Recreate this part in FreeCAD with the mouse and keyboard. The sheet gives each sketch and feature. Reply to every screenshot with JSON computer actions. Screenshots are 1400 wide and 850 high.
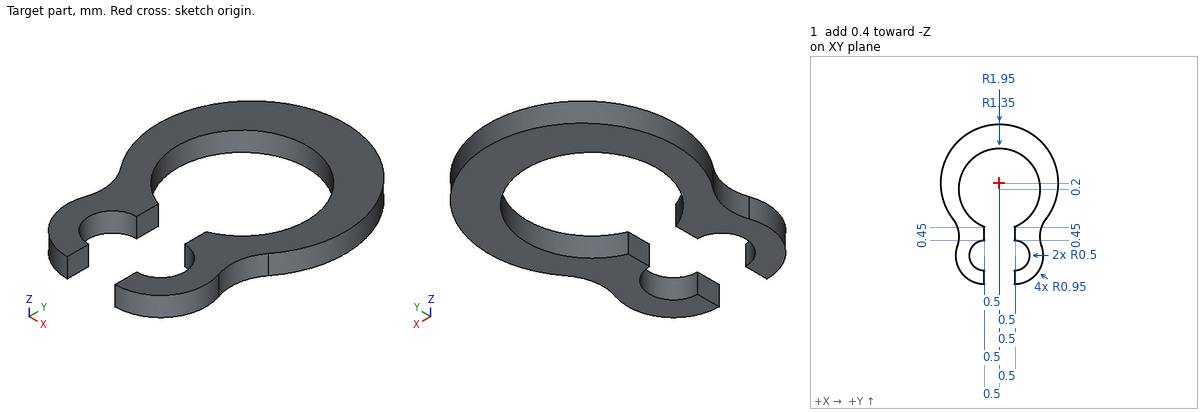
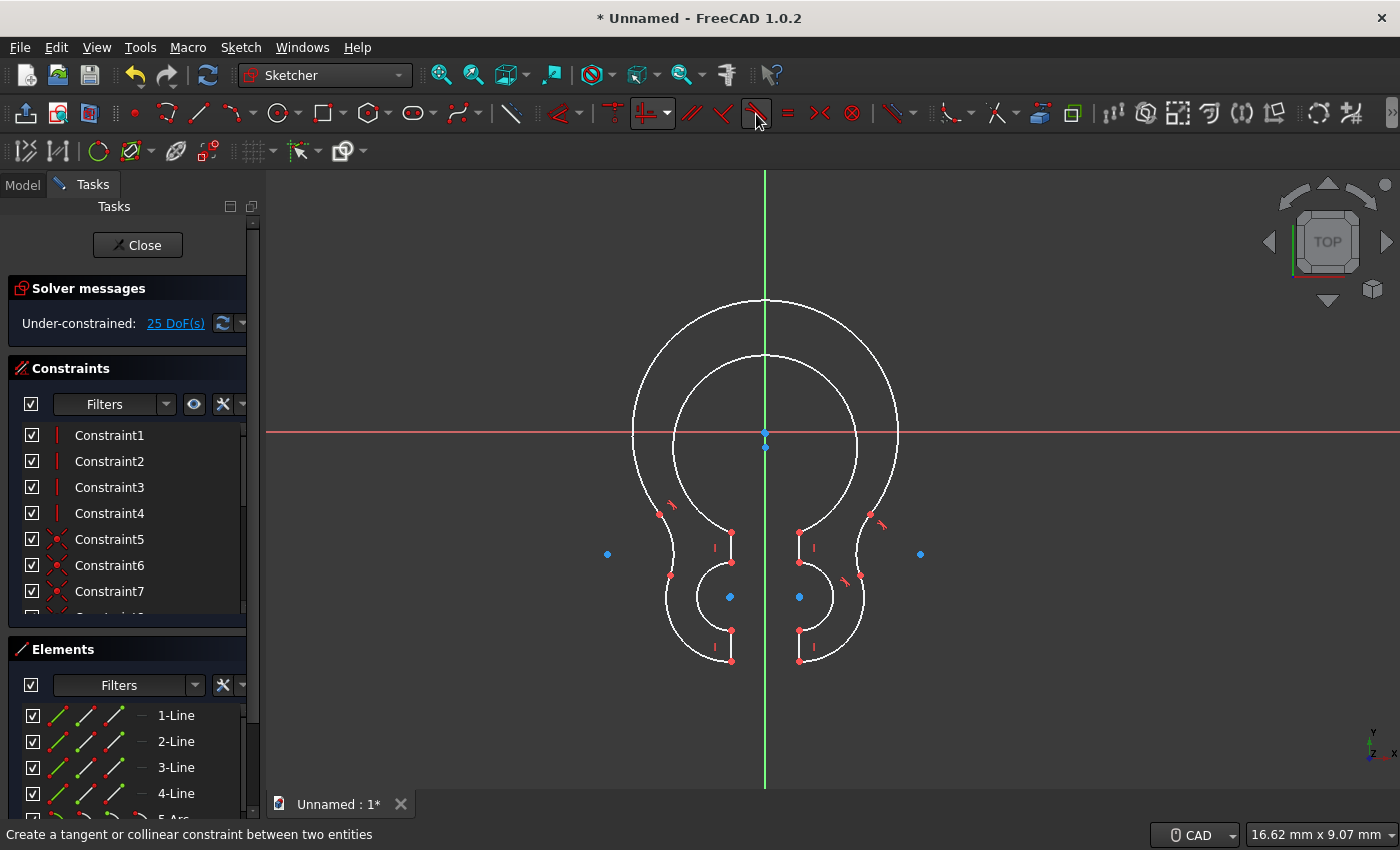
{"action": "left_click", "coordinate": [674, 557]}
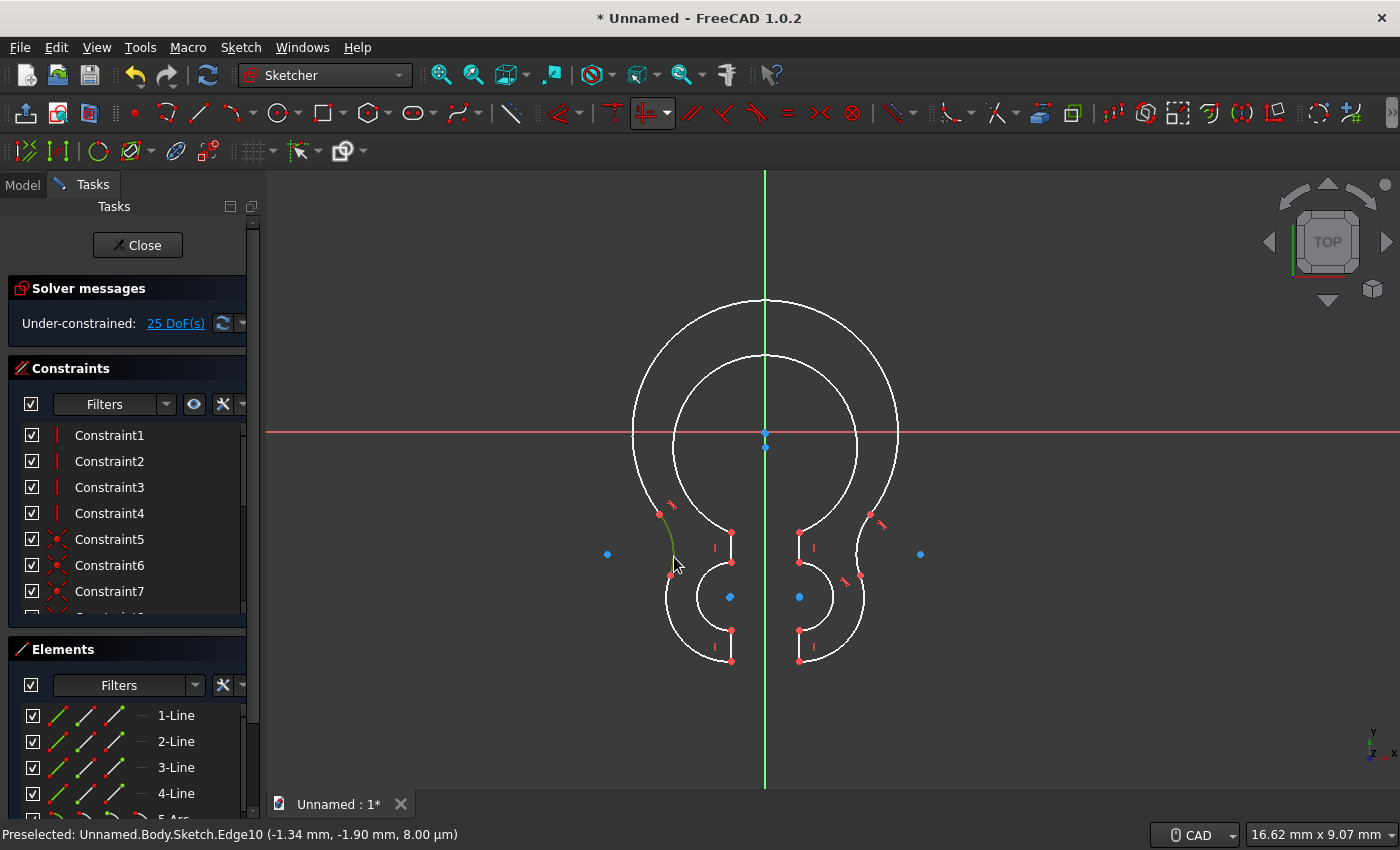
{"action": "left_click", "coordinate": [668, 613]}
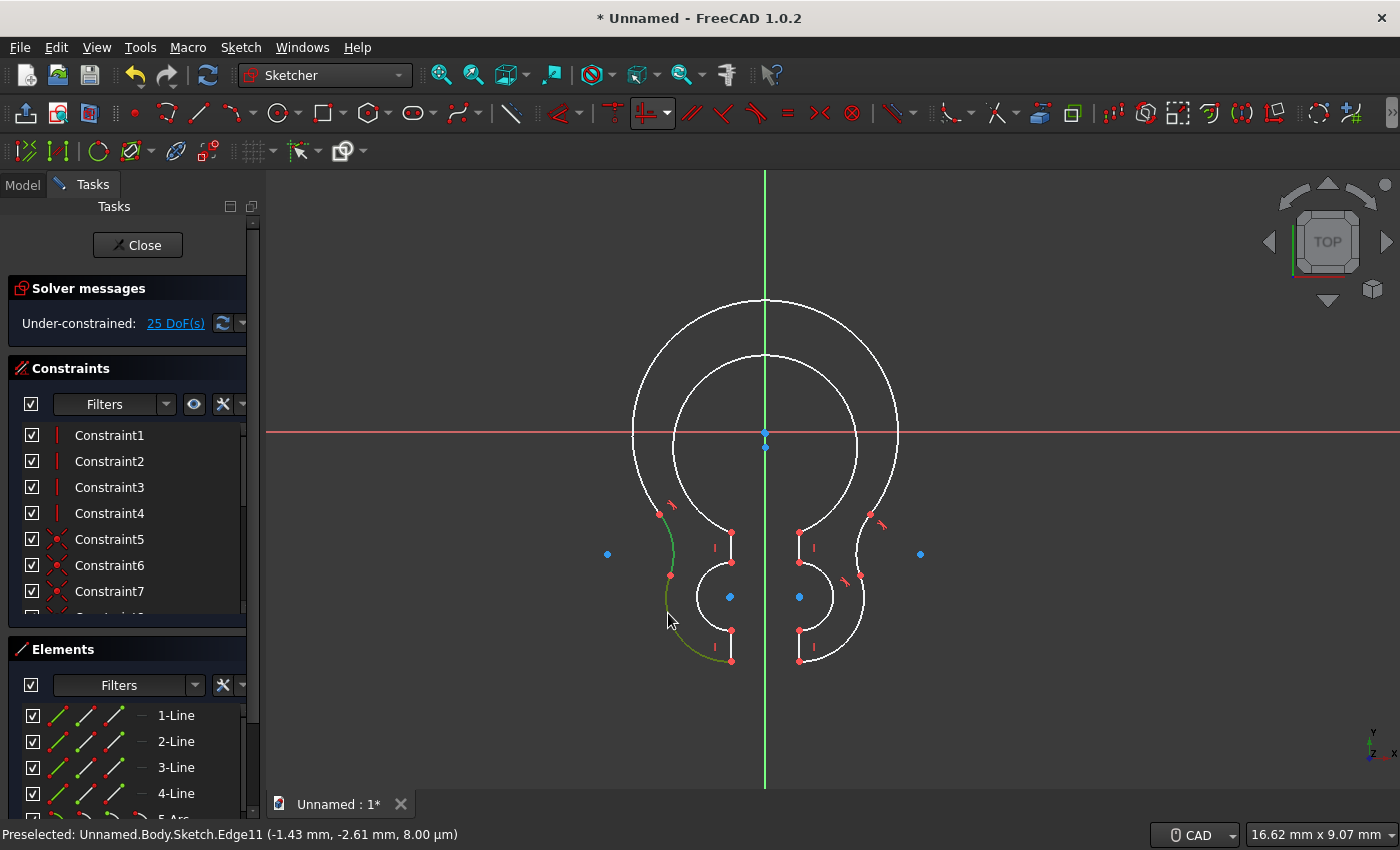
{"action": "left_click", "coordinate": [756, 114]}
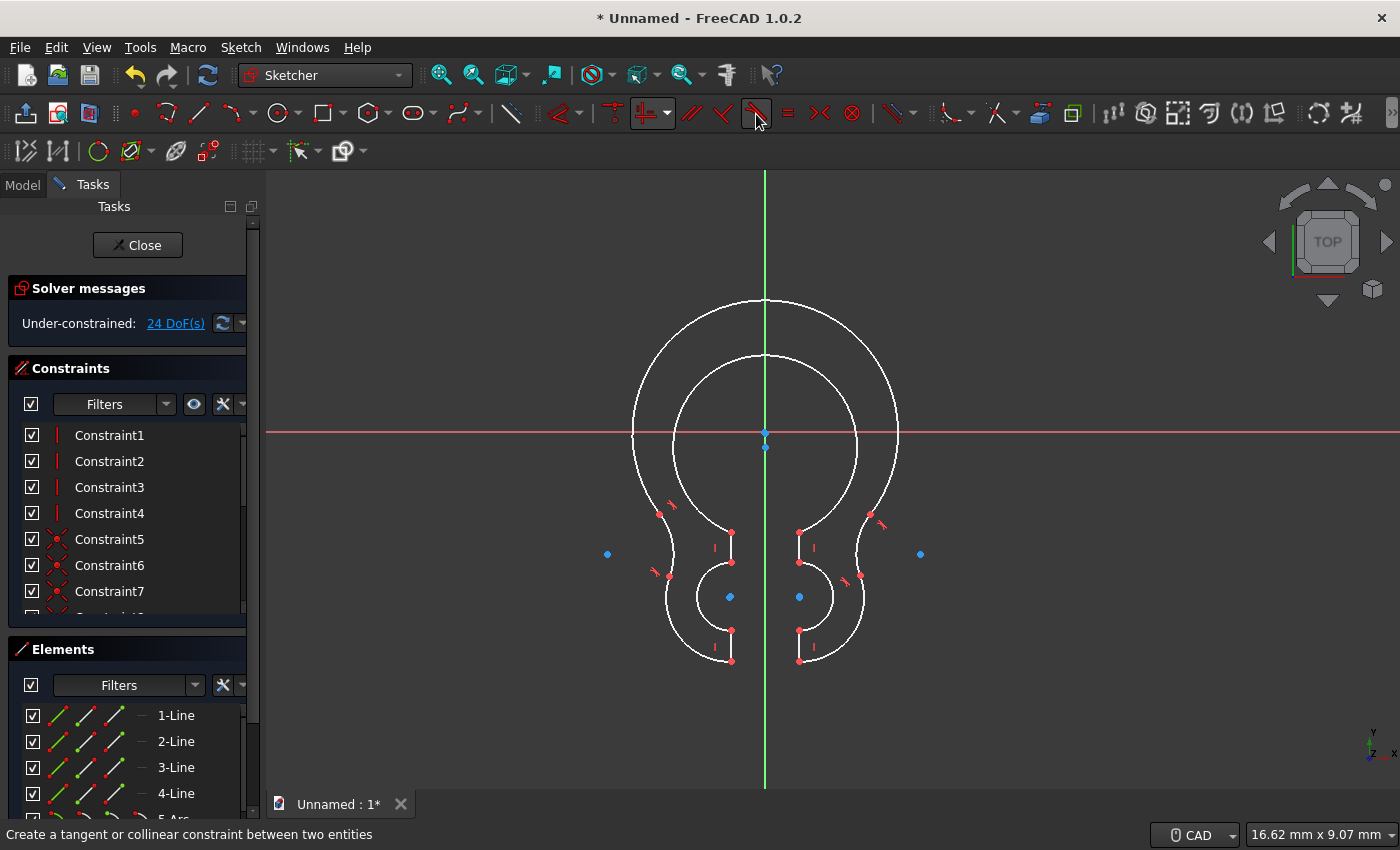
{"action": "left_click", "coordinate": [827, 617]}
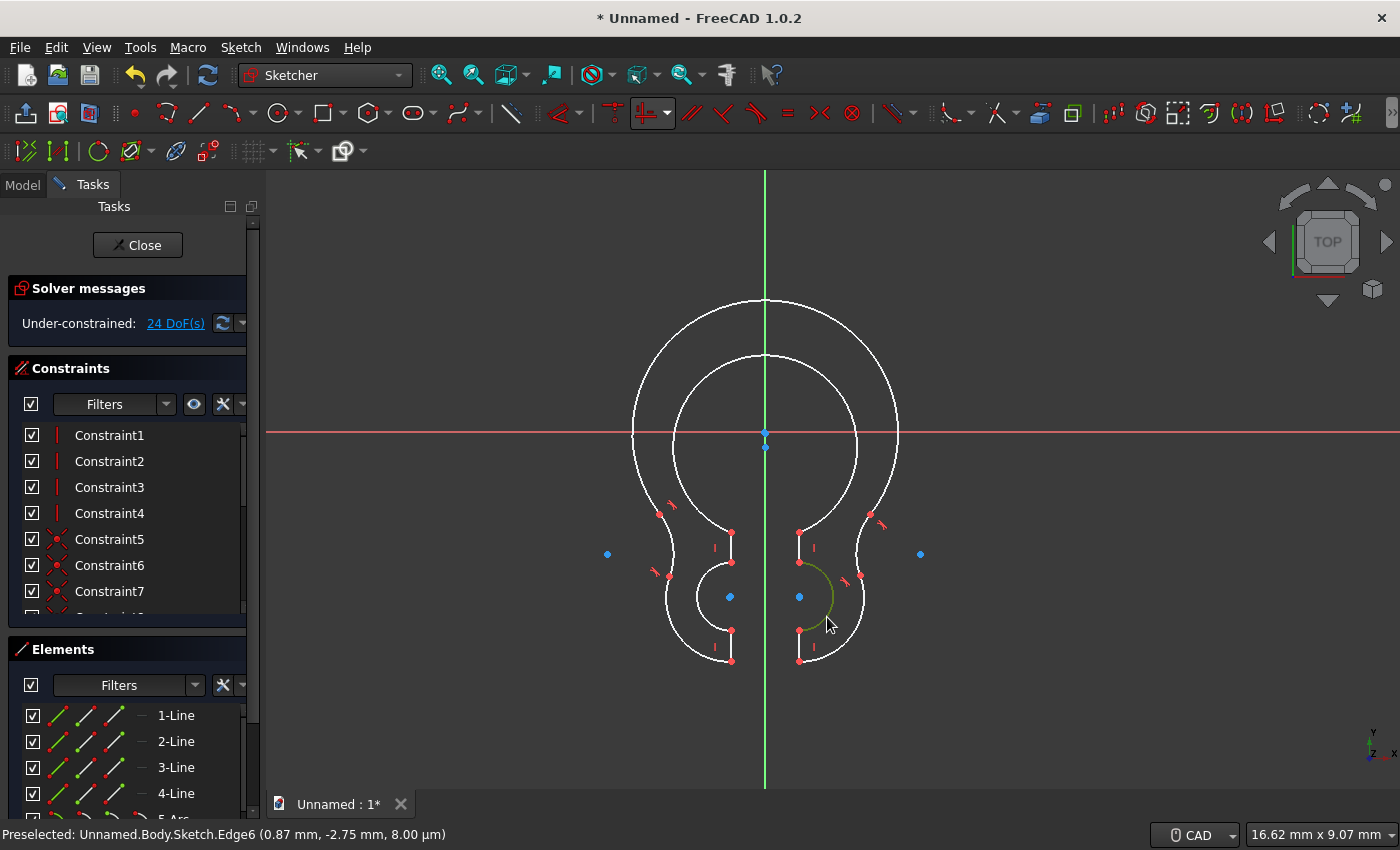
{"action": "left_click", "coordinate": [834, 652]}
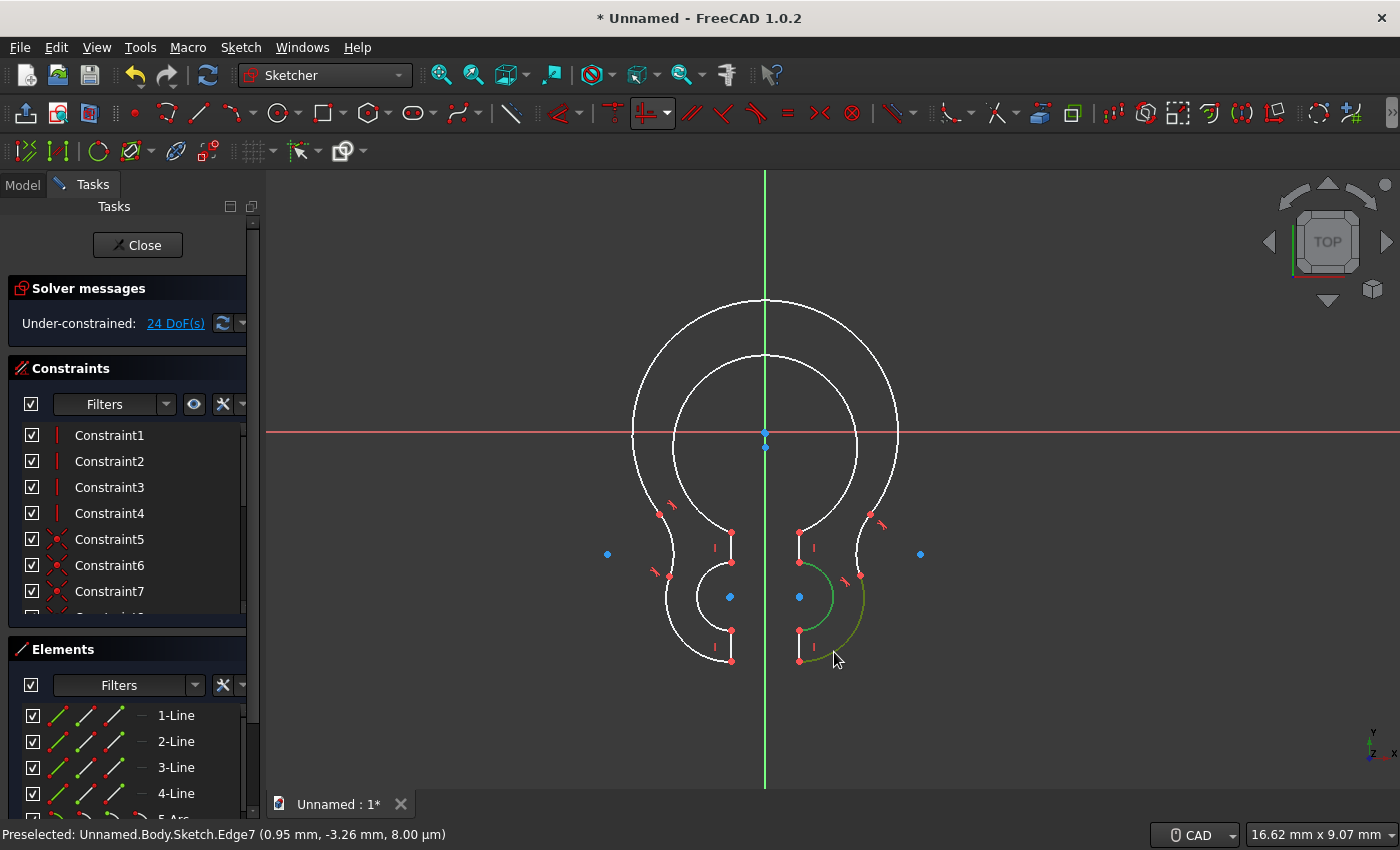
{"action": "key", "text": "c"}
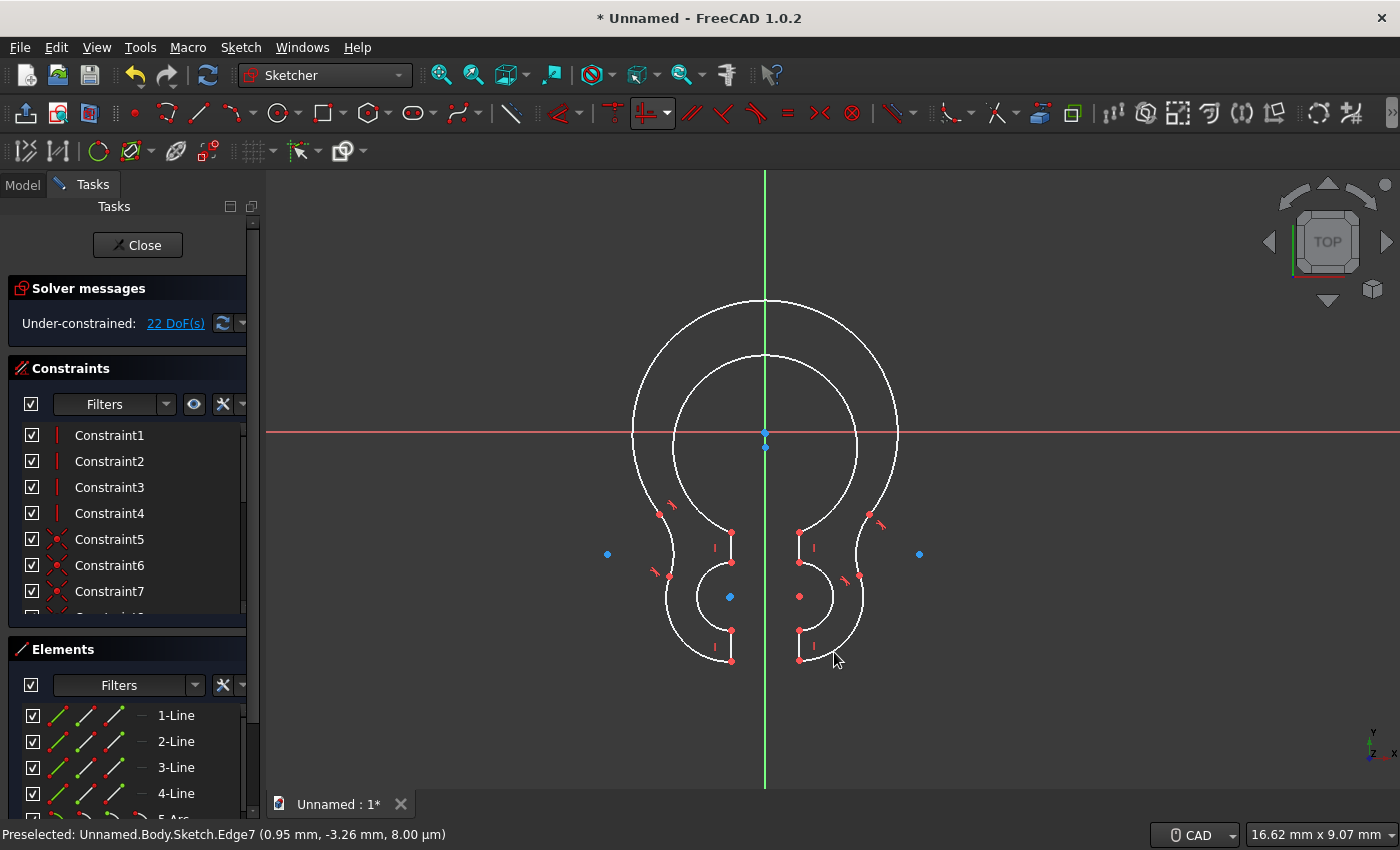
{"action": "left_click", "coordinate": [668, 613]}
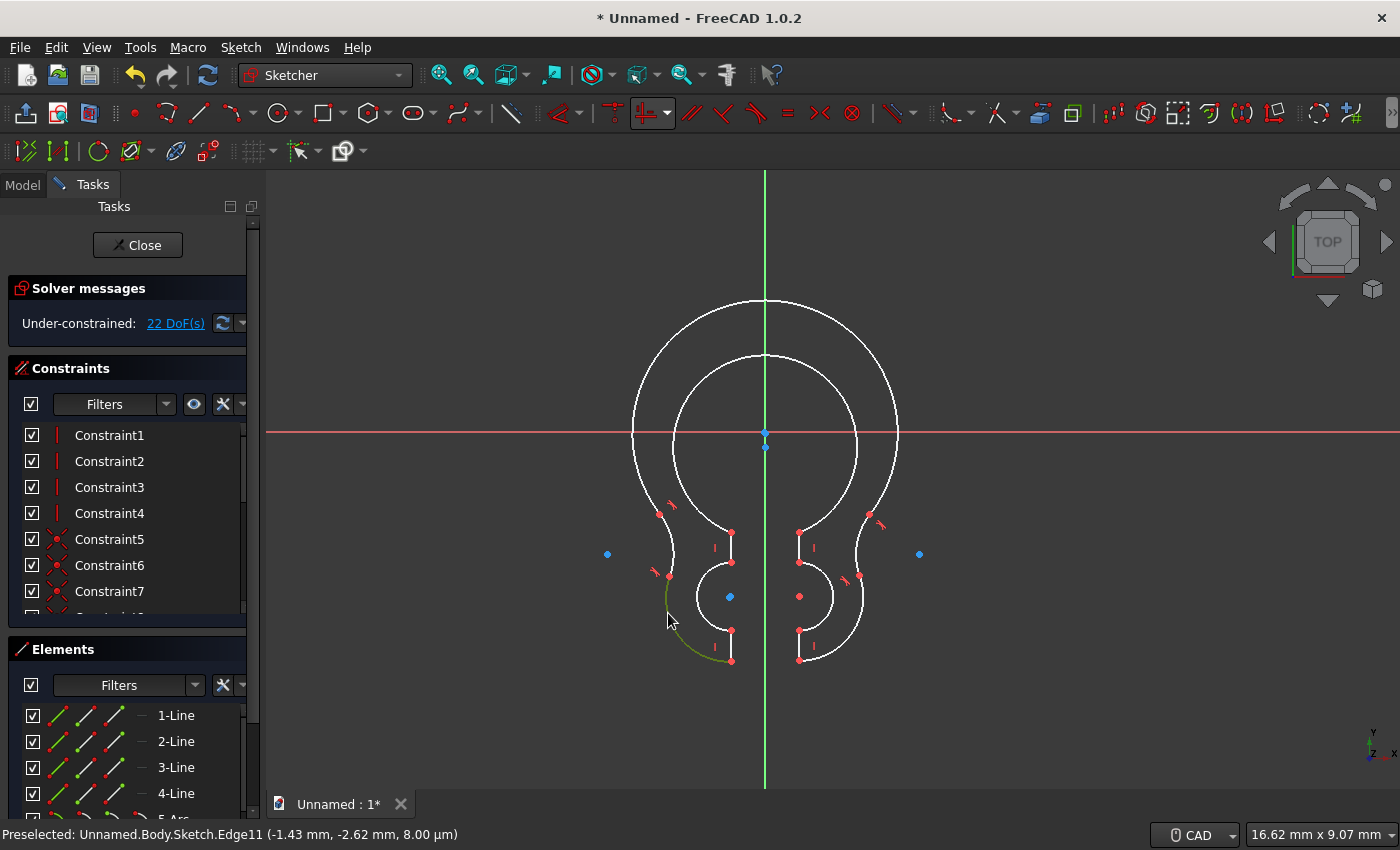
{"action": "left_click", "coordinate": [704, 577]}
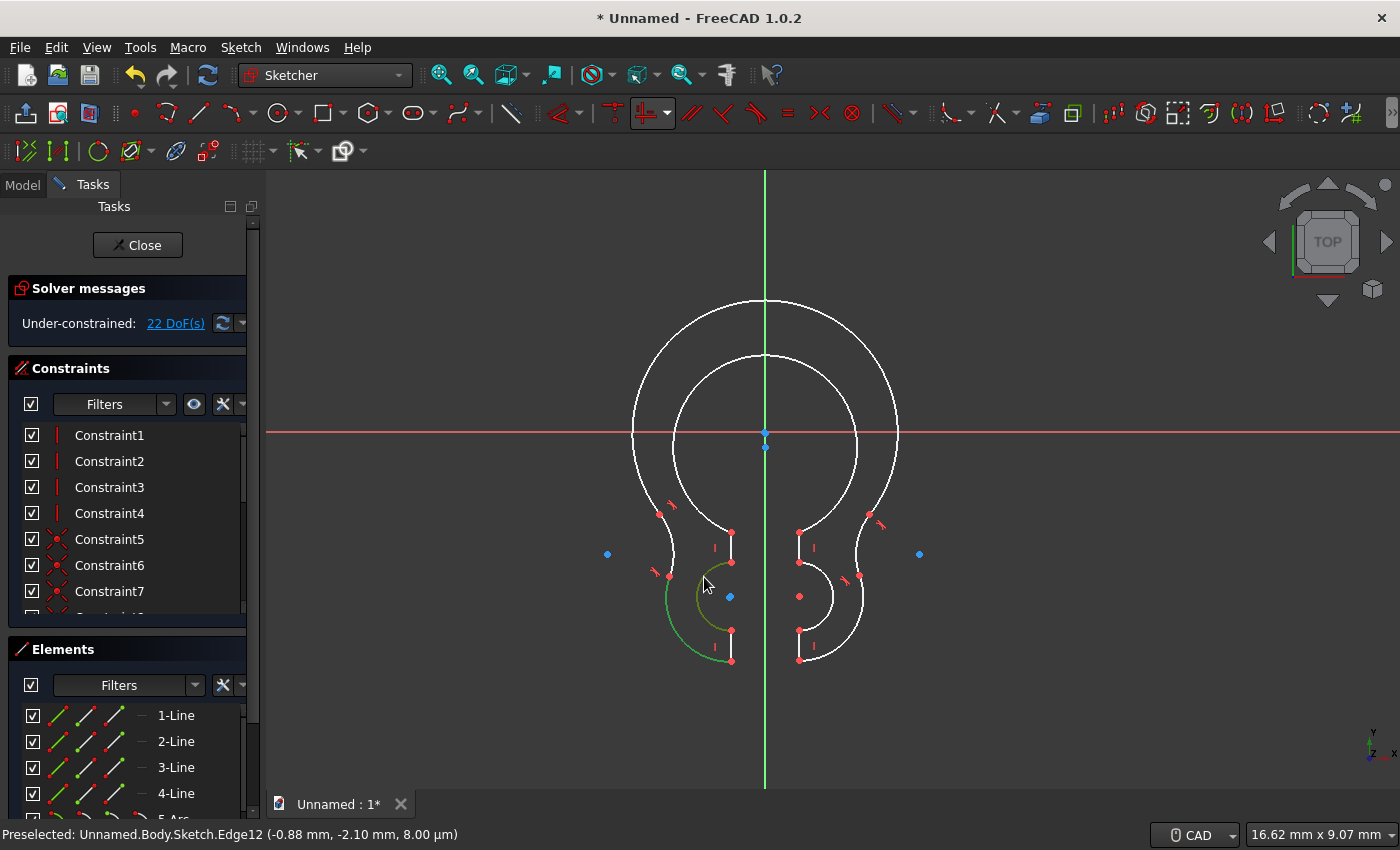
{"action": "key", "text": "c"}